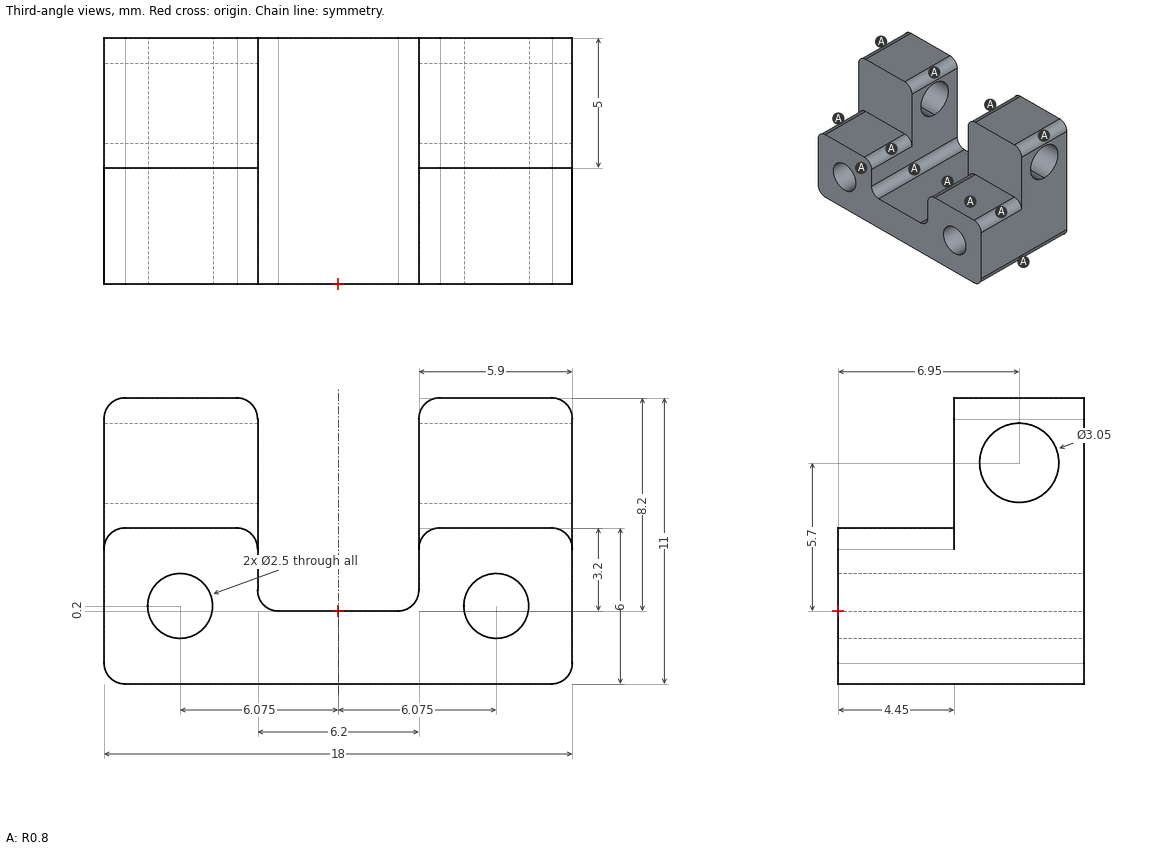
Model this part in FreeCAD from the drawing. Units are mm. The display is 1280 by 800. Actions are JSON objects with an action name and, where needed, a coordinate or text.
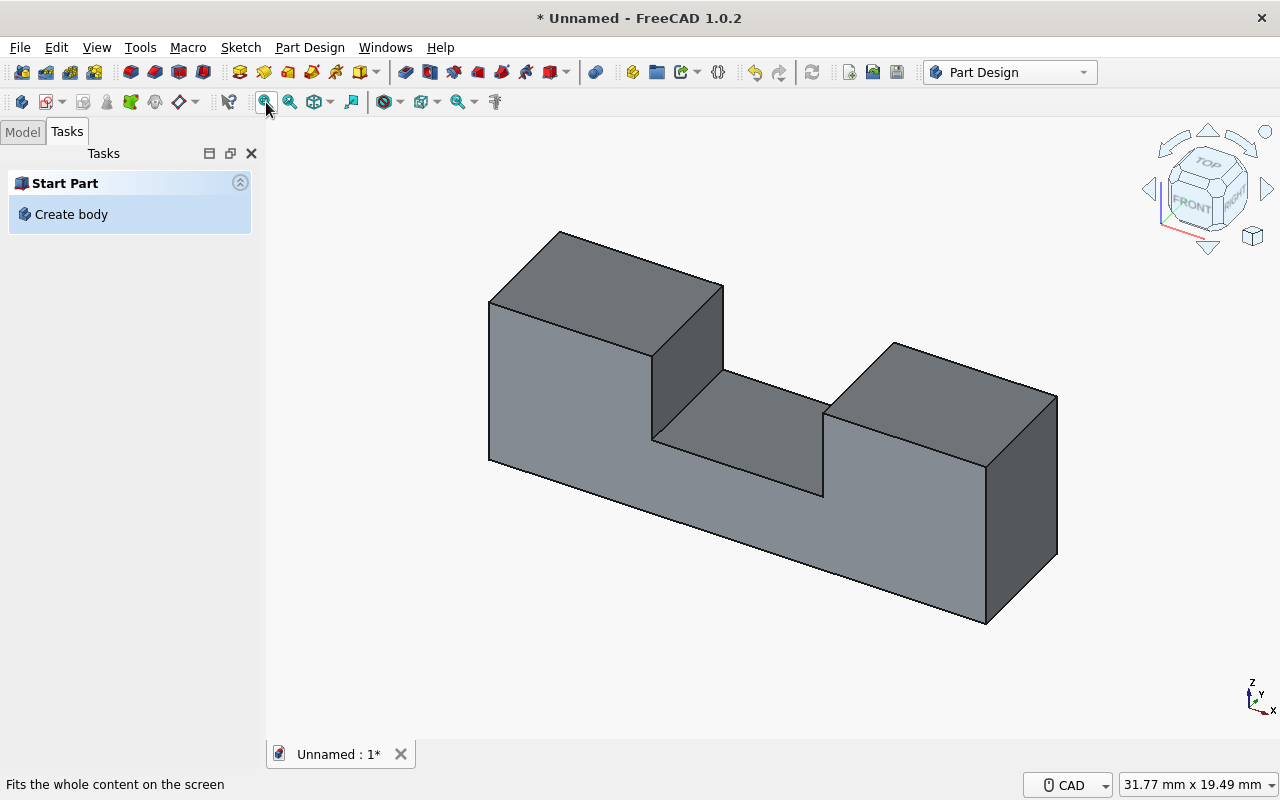
{"action": "key", "text": "4"}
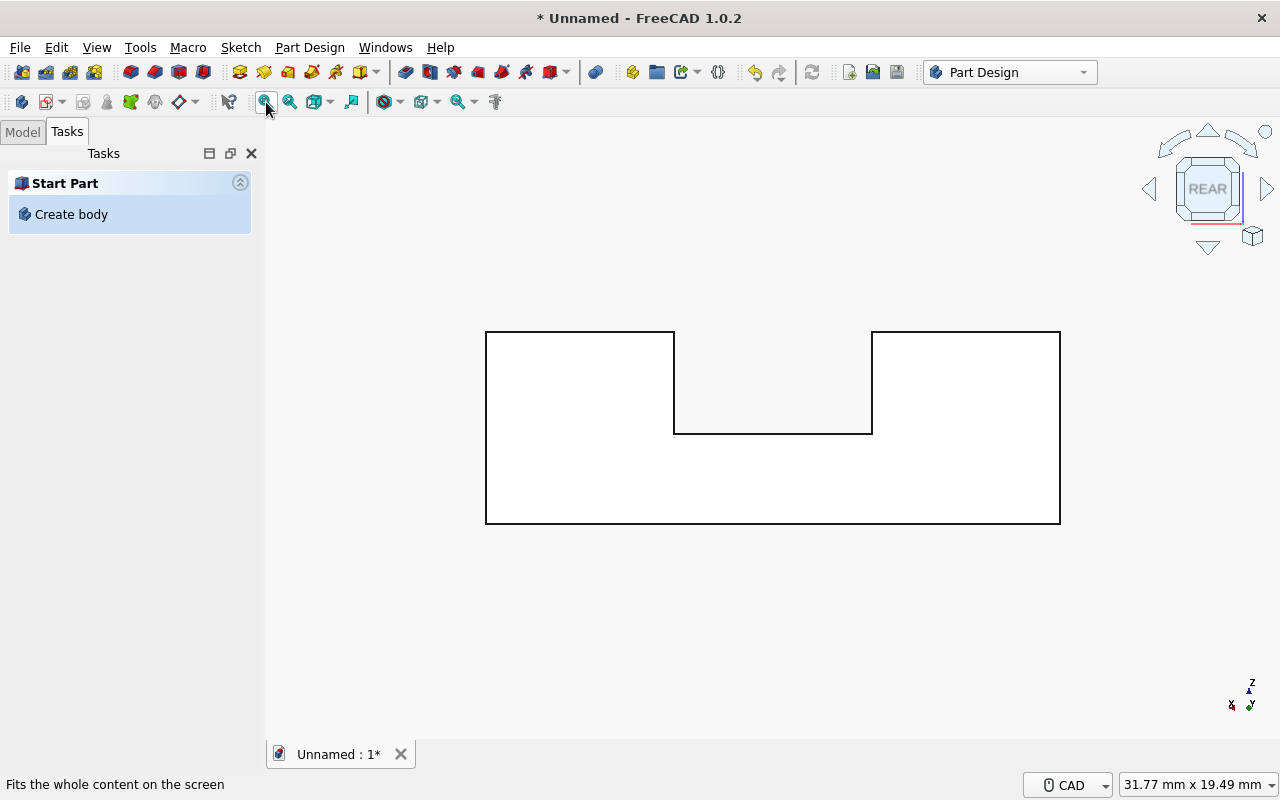
{"action": "left_click", "coordinate": [609, 454]}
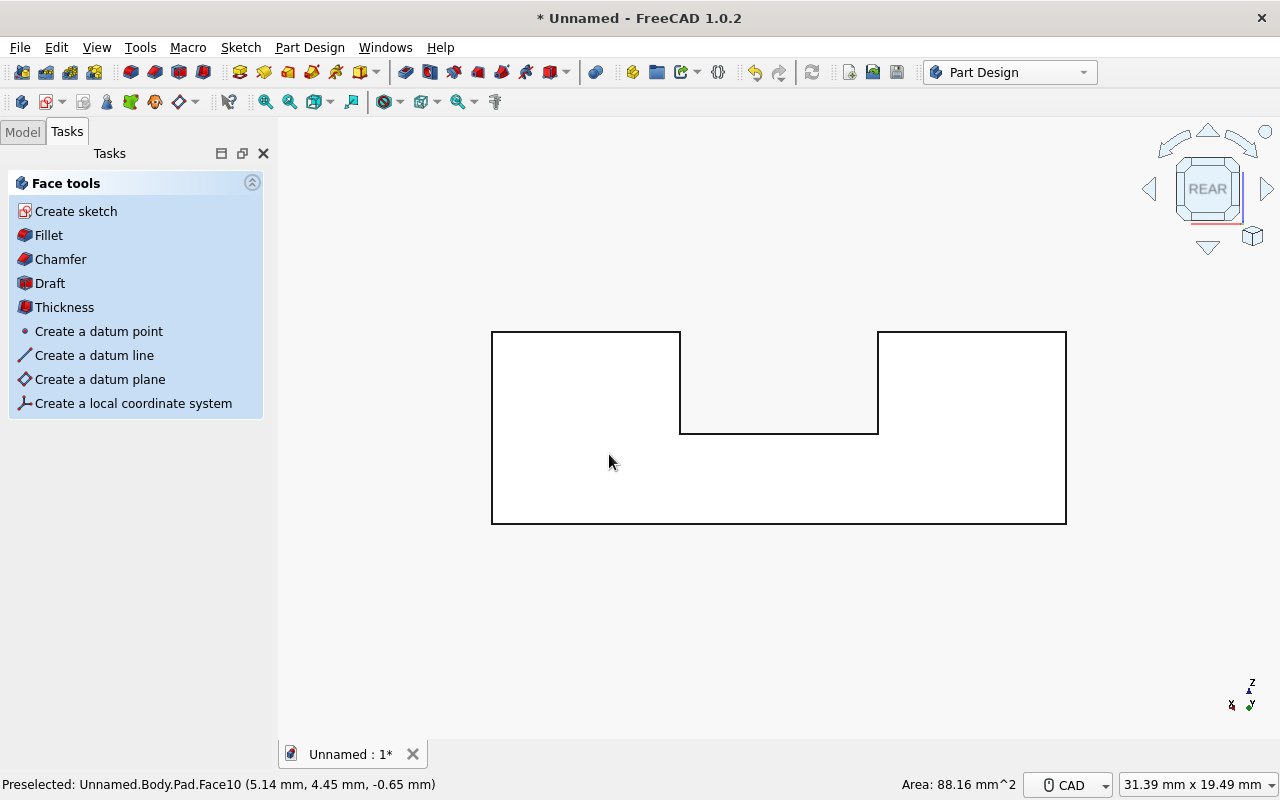
{"action": "left_click", "coordinate": [46, 102]}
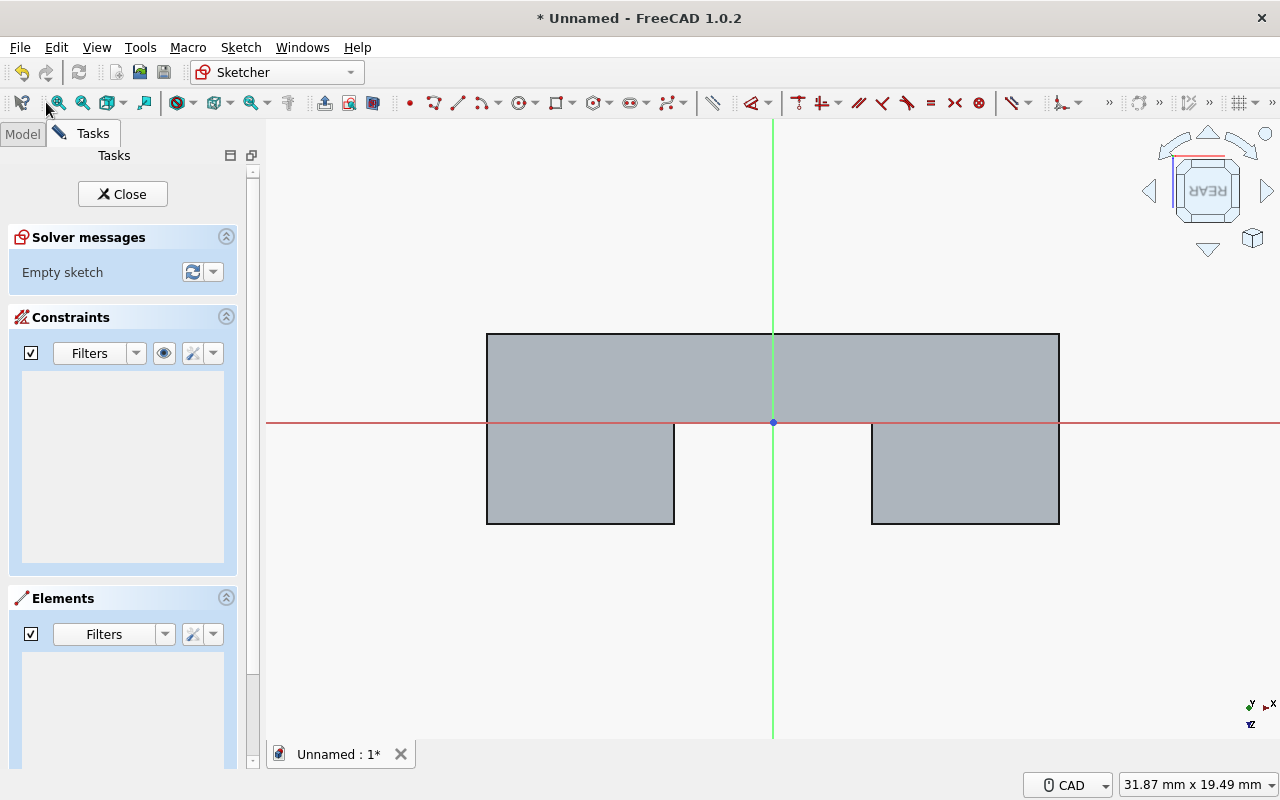
{"action": "left_click", "coordinate": [434, 104]}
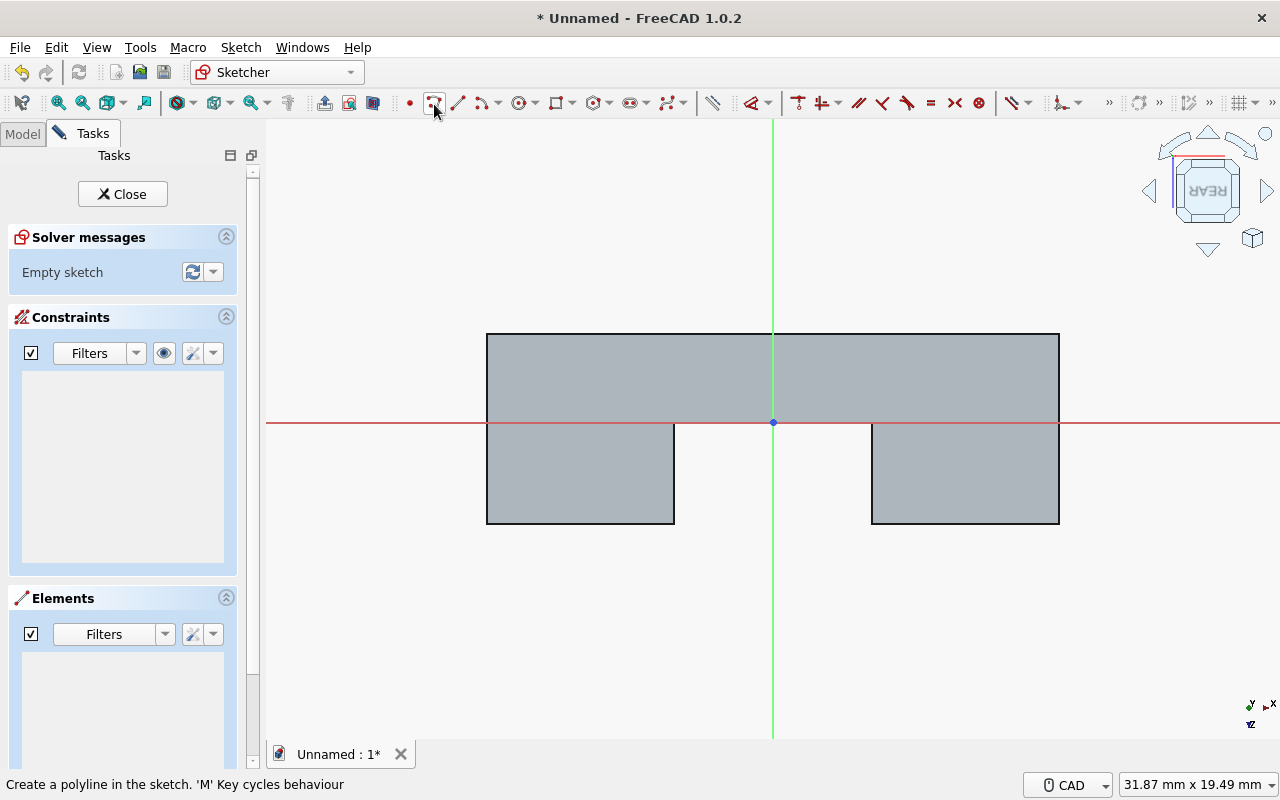
{"action": "left_click", "coordinate": [674, 423]}
{"action": "left_click", "coordinate": [872, 432]}
{"action": "left_click", "coordinate": [872, 684]}
{"action": "left_click", "coordinate": [1059, 684]}
{"action": "left_click", "coordinate": [1059, 334]}
{"action": "left_click", "coordinate": [487, 334]}
{"action": "left_click", "coordinate": [487, 684]}
{"action": "left_click", "coordinate": [674, 684]}
{"action": "left_click", "coordinate": [674, 423]}
{"action": "key", "text": "Escape"}
{"action": "key", "text": "Escape"}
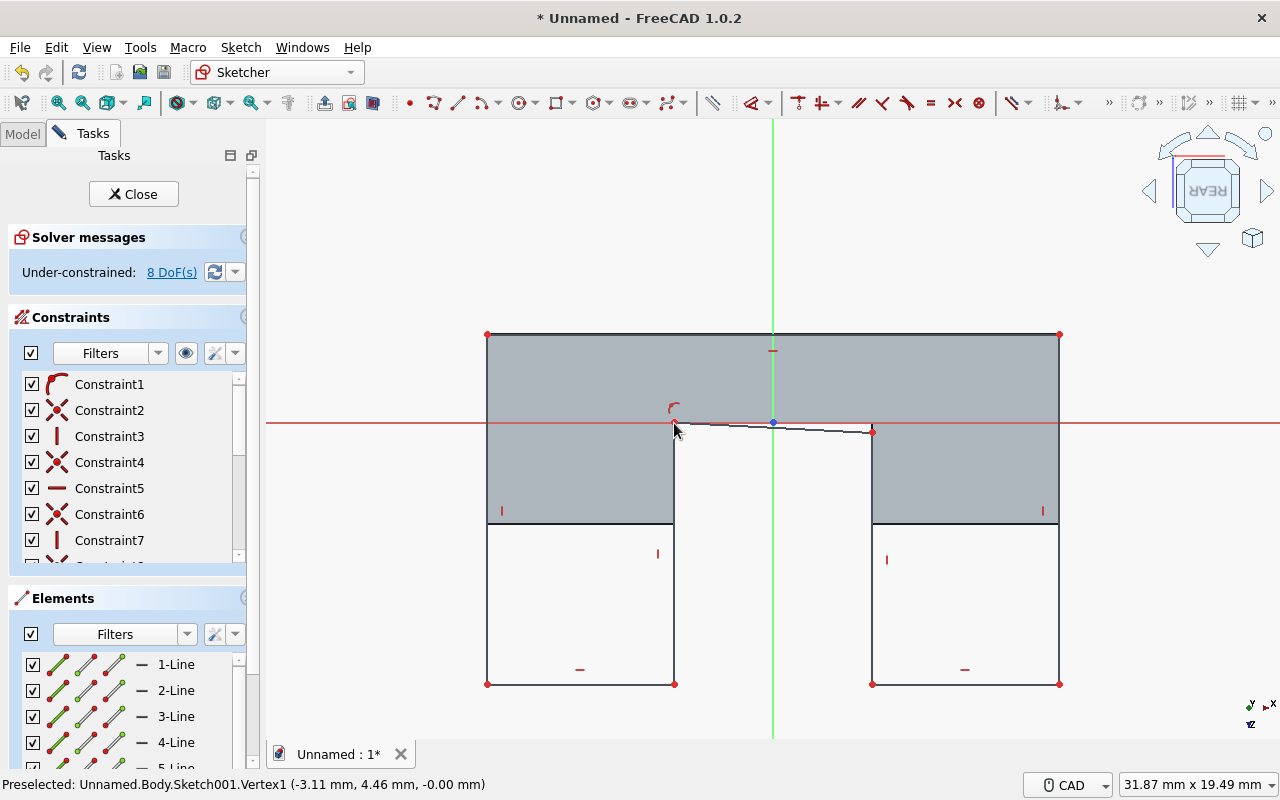
{"action": "left_click", "coordinate": [733, 426]}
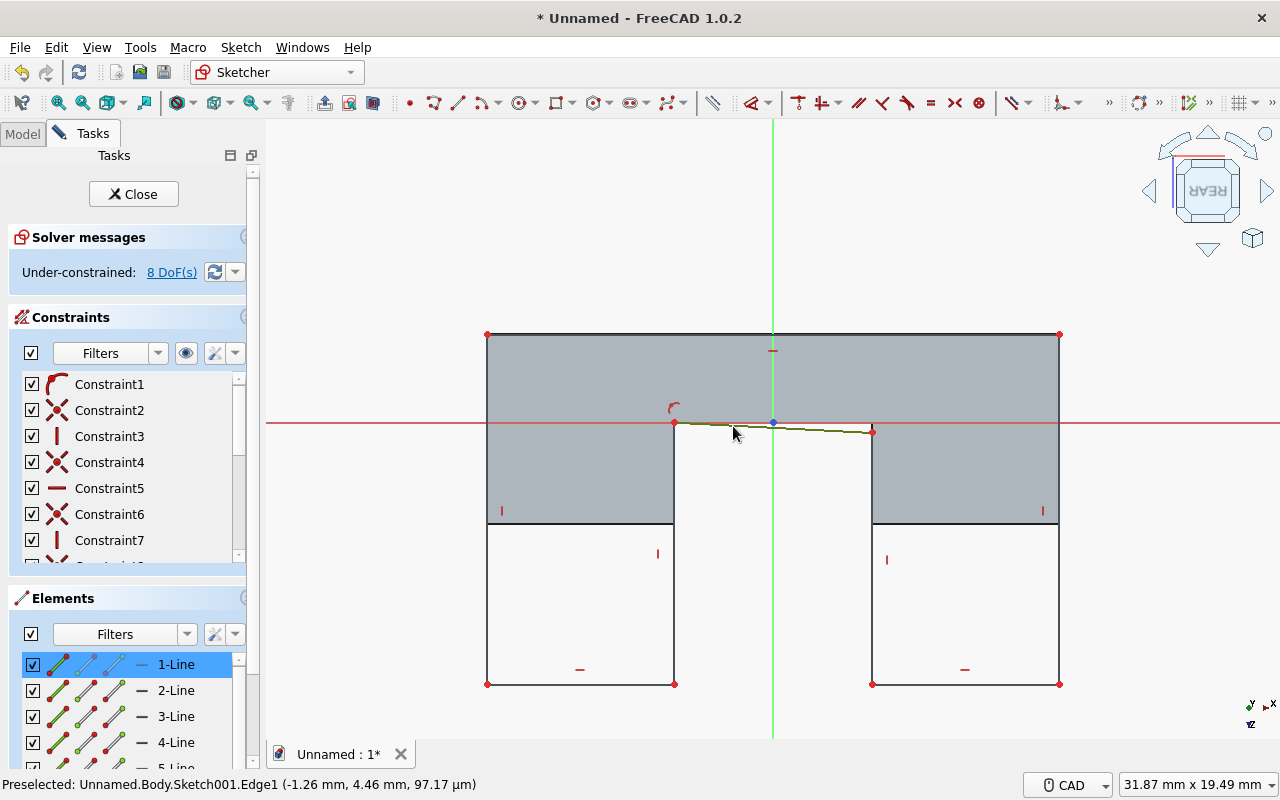
{"action": "left_click", "coordinate": [840, 104]}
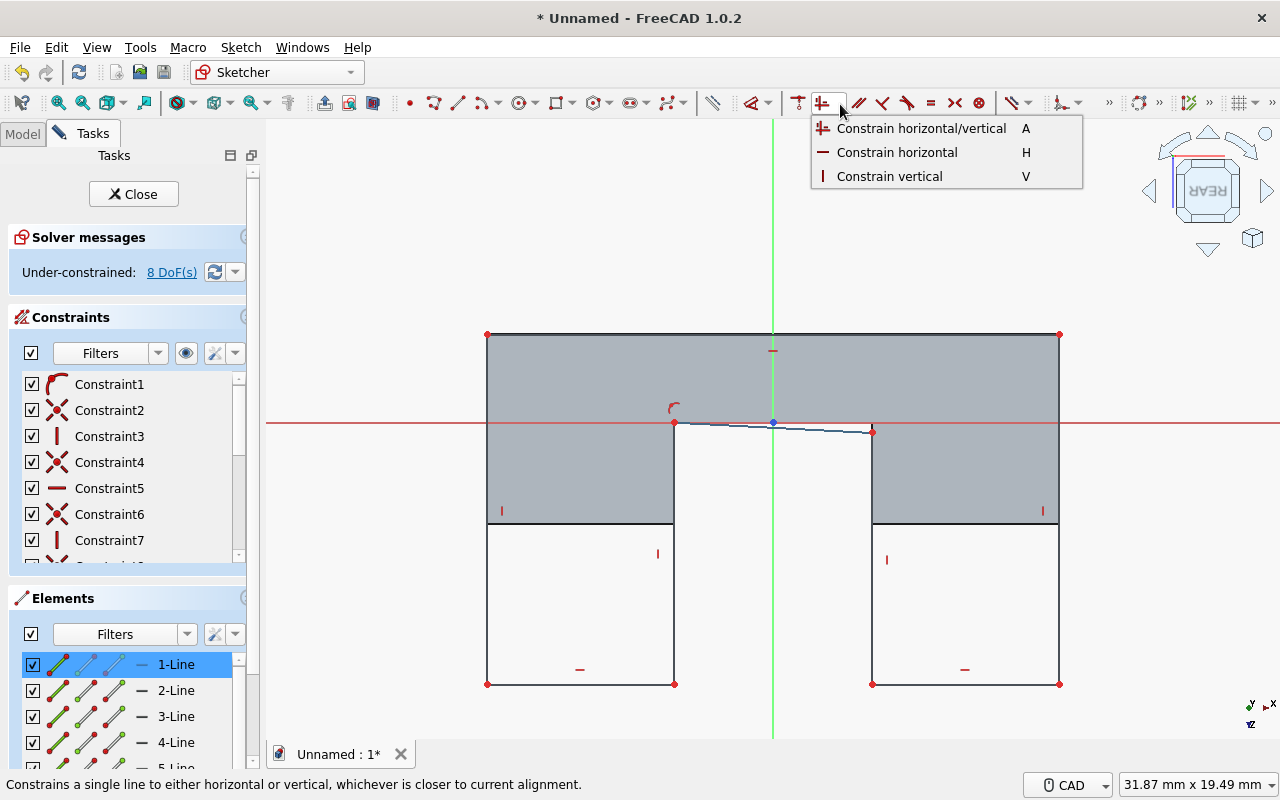
{"action": "left_click", "coordinate": [947, 152]}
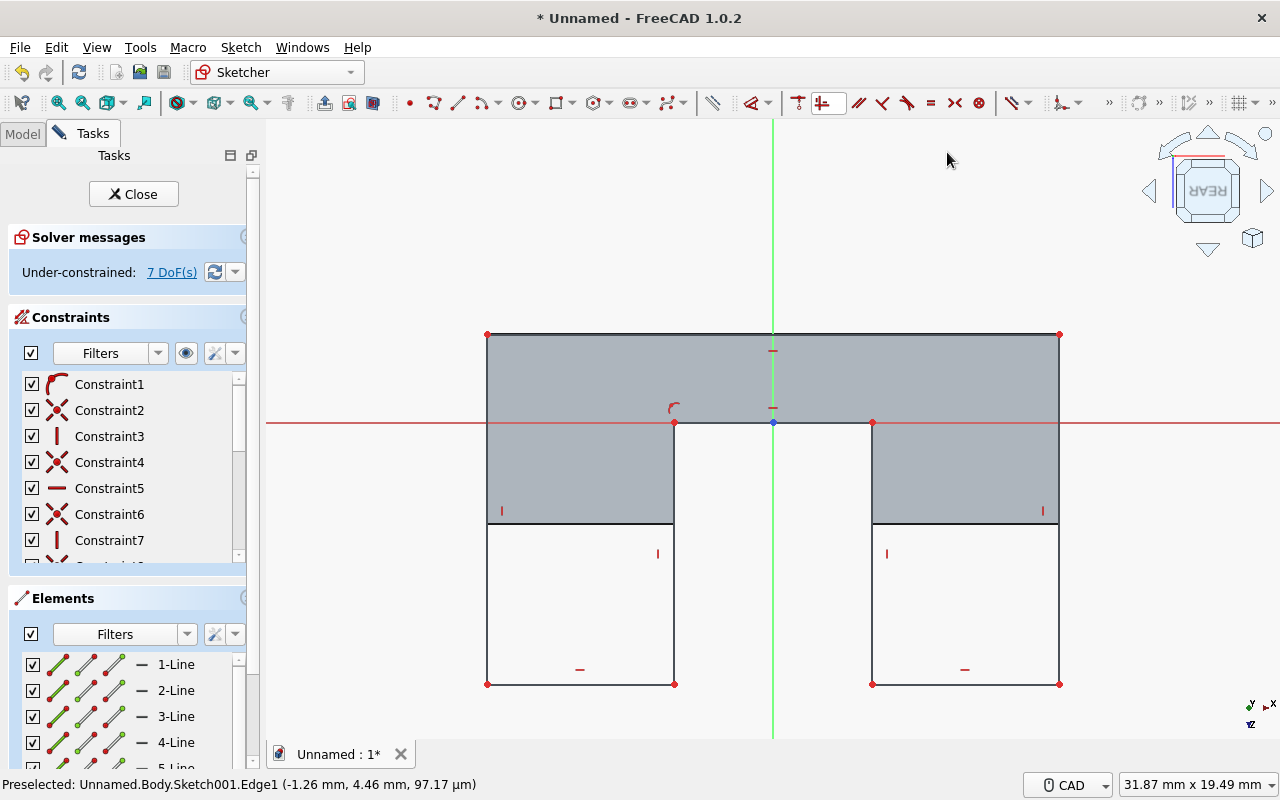
{"action": "left_click", "coordinate": [1059, 685]}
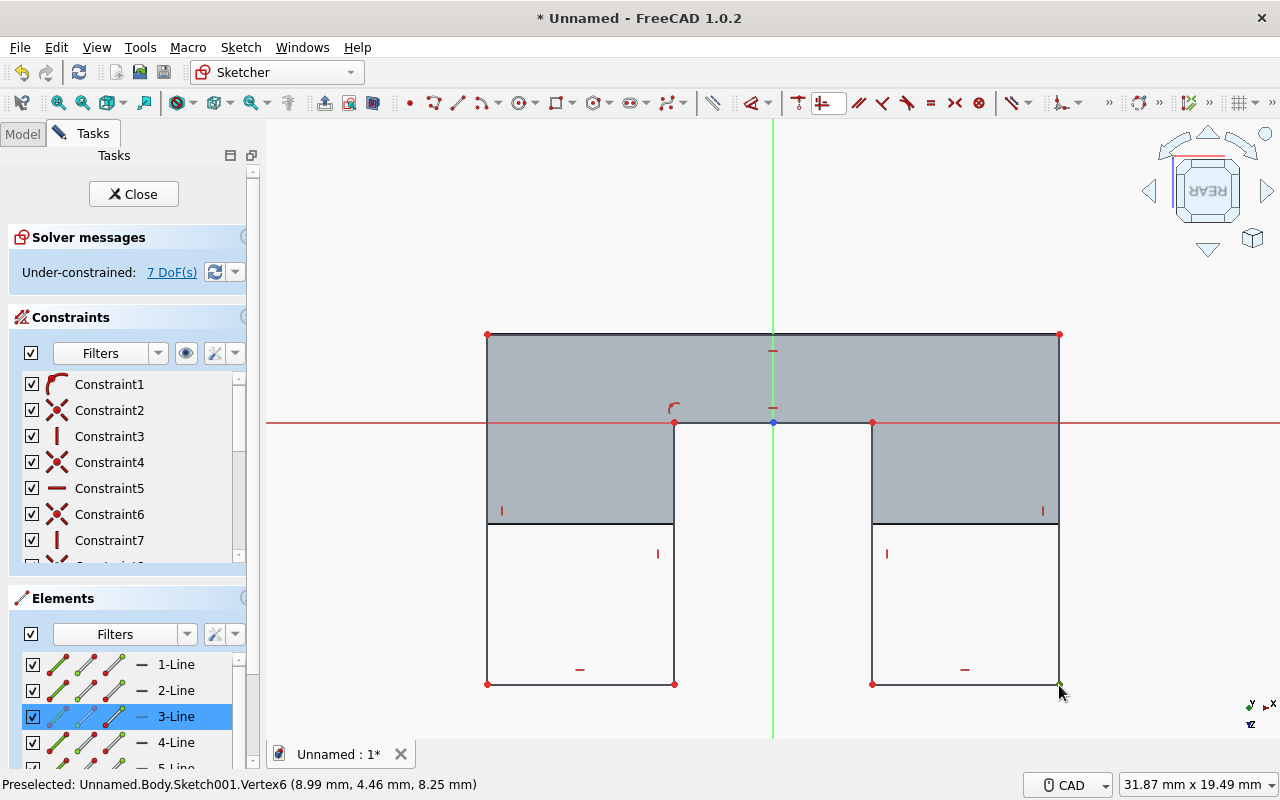
{"action": "left_click", "coordinate": [487, 685]}